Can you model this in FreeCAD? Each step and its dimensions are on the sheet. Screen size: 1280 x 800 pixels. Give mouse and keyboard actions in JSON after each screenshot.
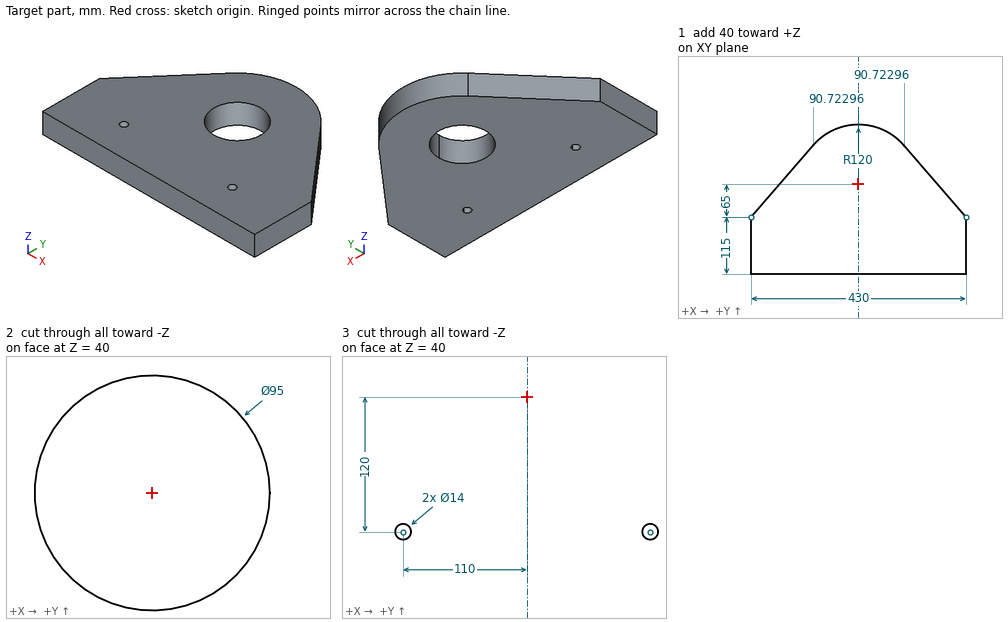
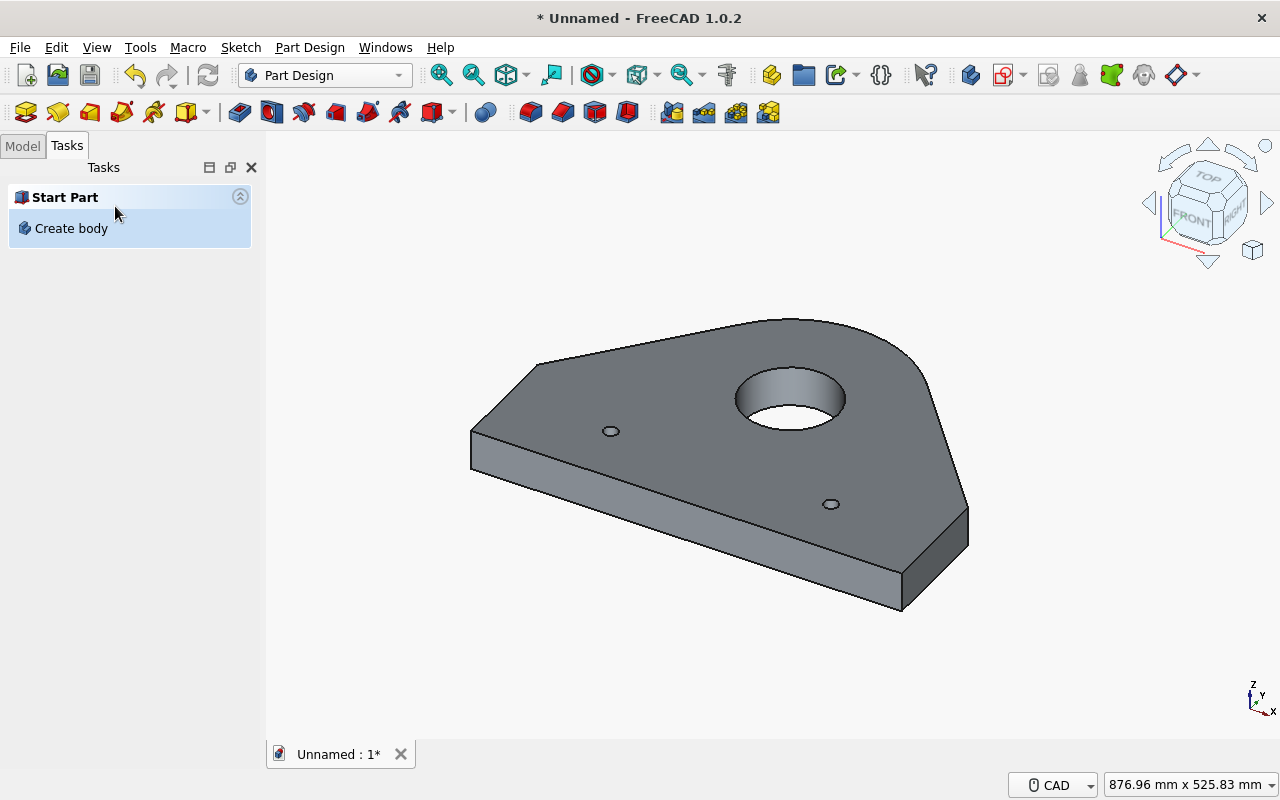
{"action": "key", "text": "0"}